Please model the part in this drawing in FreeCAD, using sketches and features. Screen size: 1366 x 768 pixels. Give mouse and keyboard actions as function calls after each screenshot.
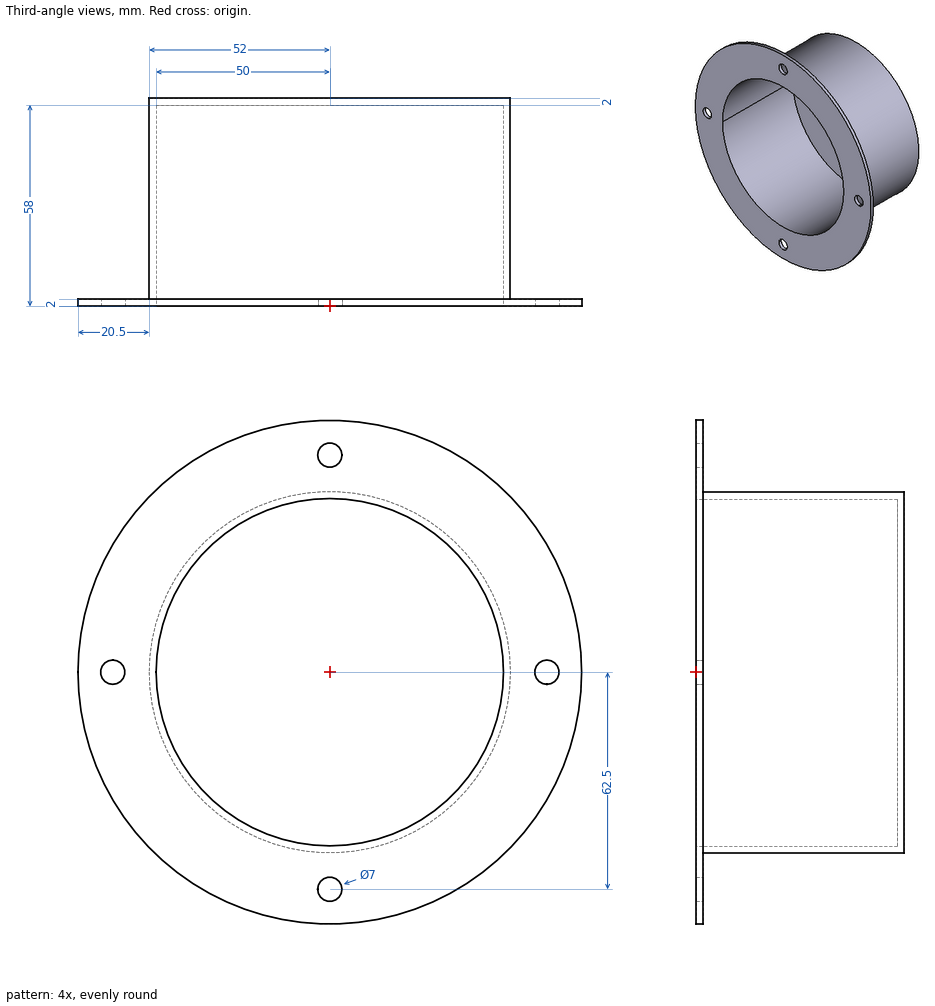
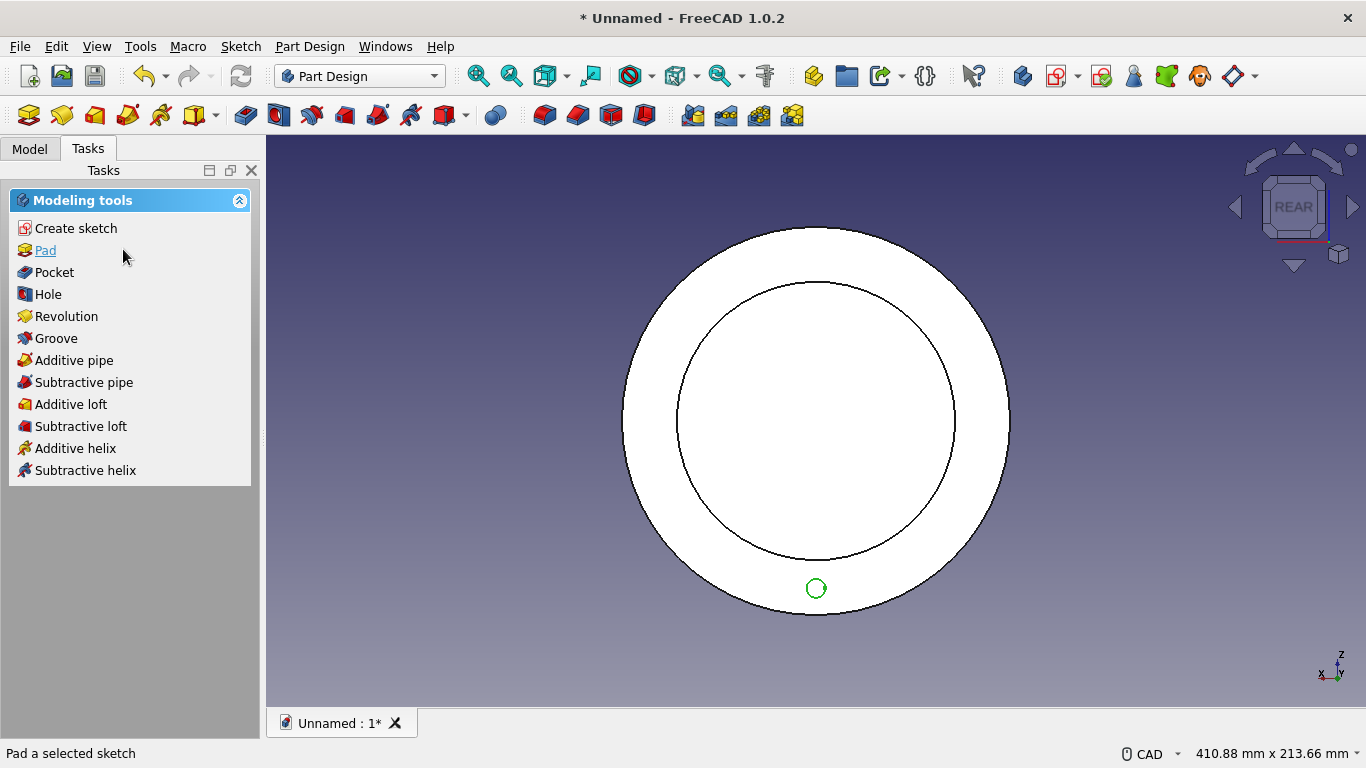
click(246, 116)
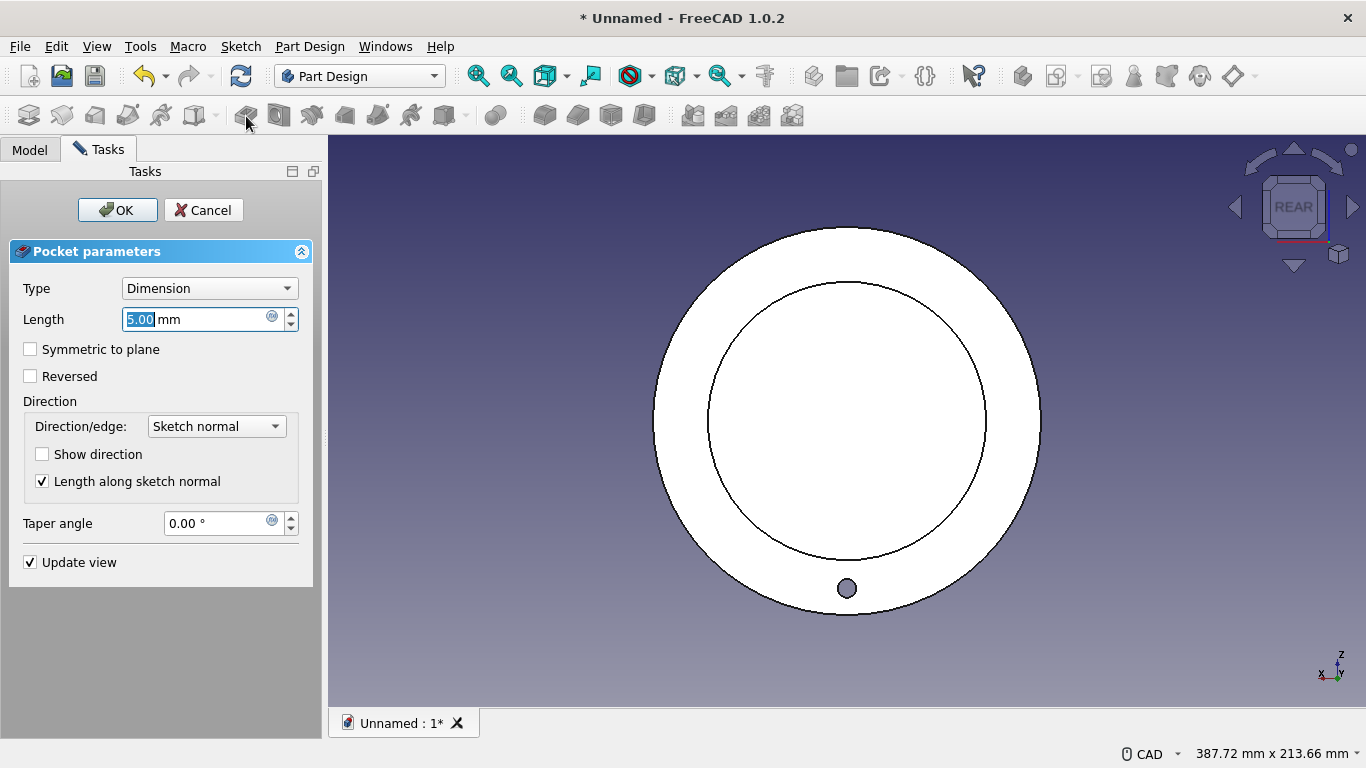
click(210, 288)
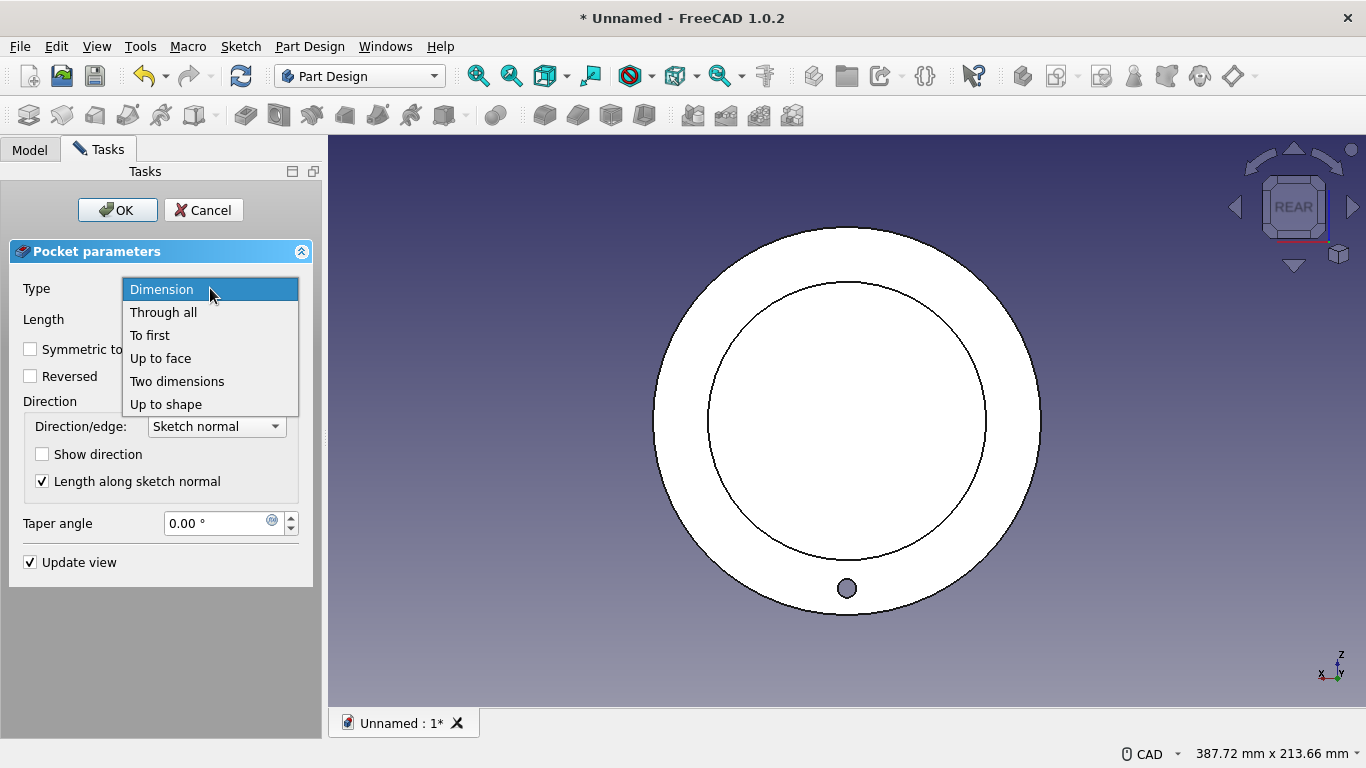
click(208, 312)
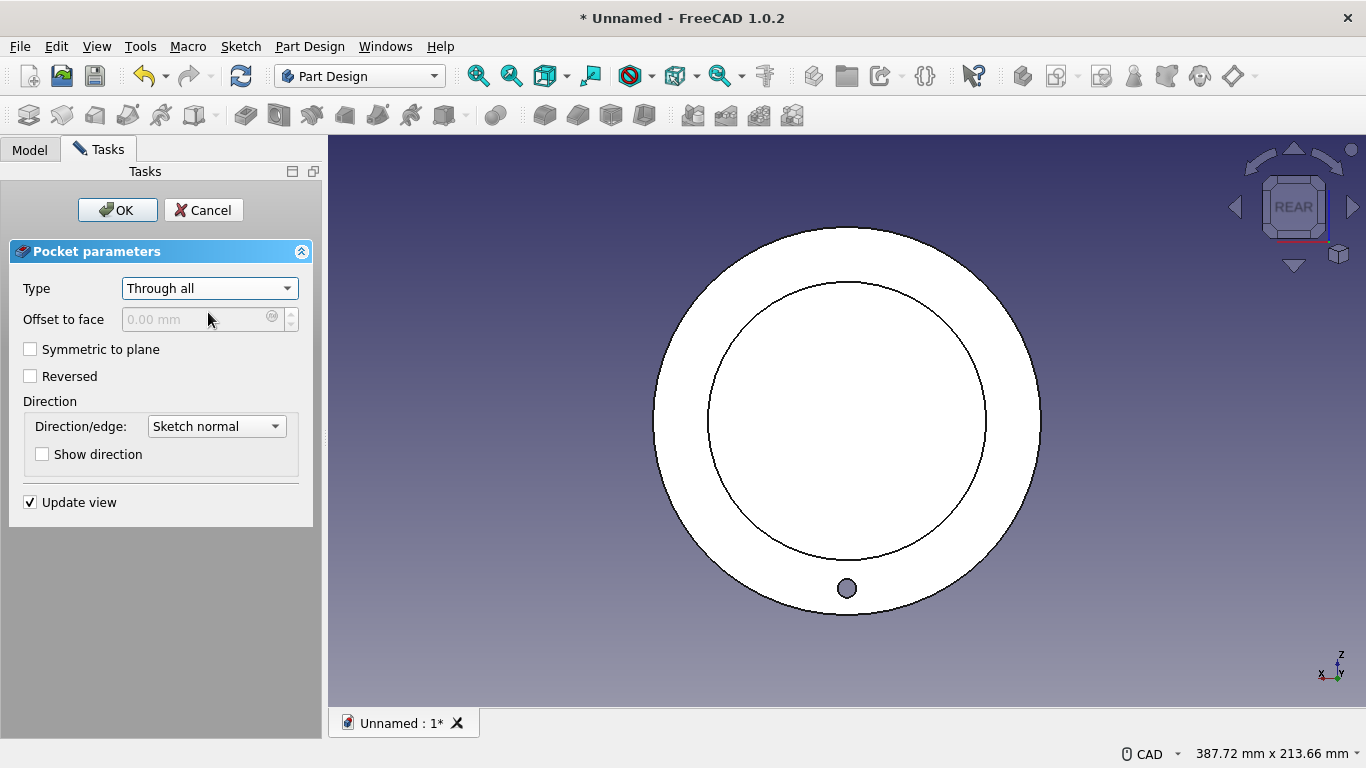
click(118, 210)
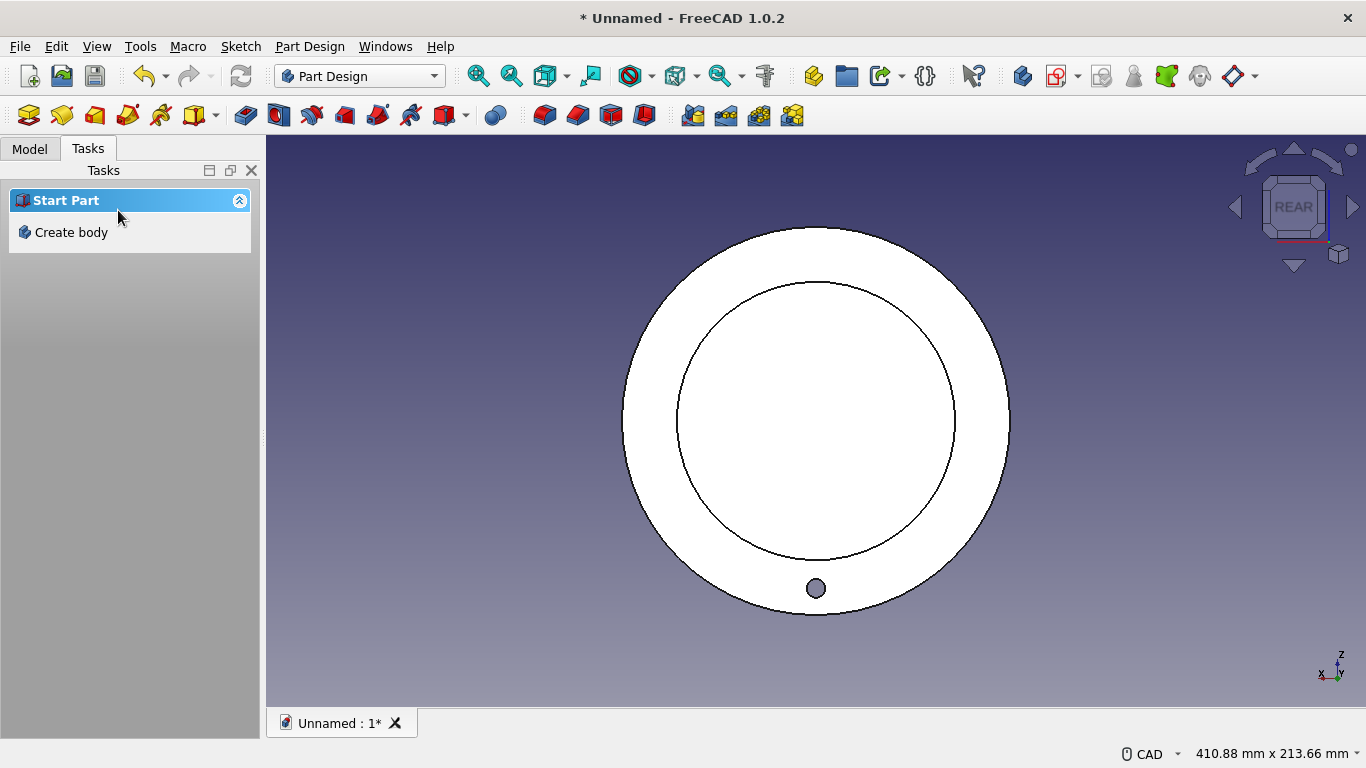
click(30, 148)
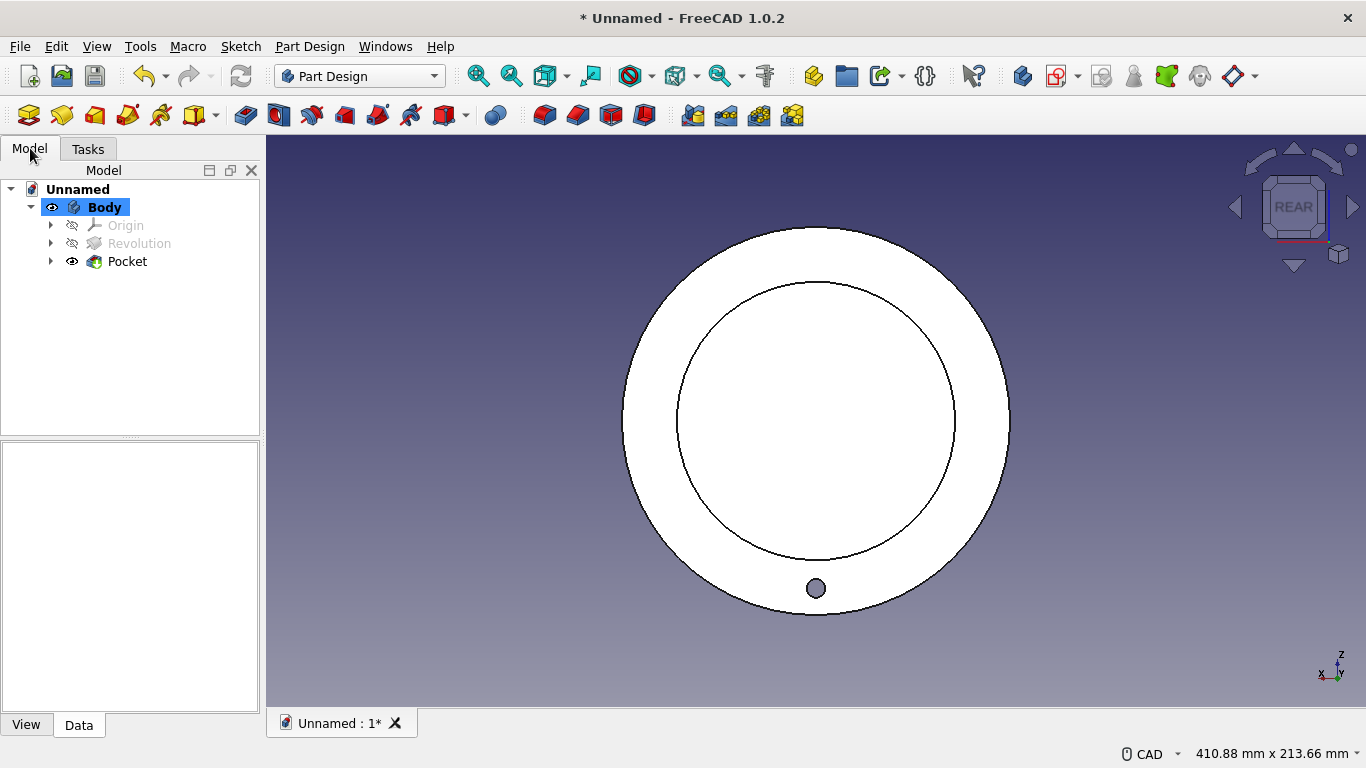
click(117, 261)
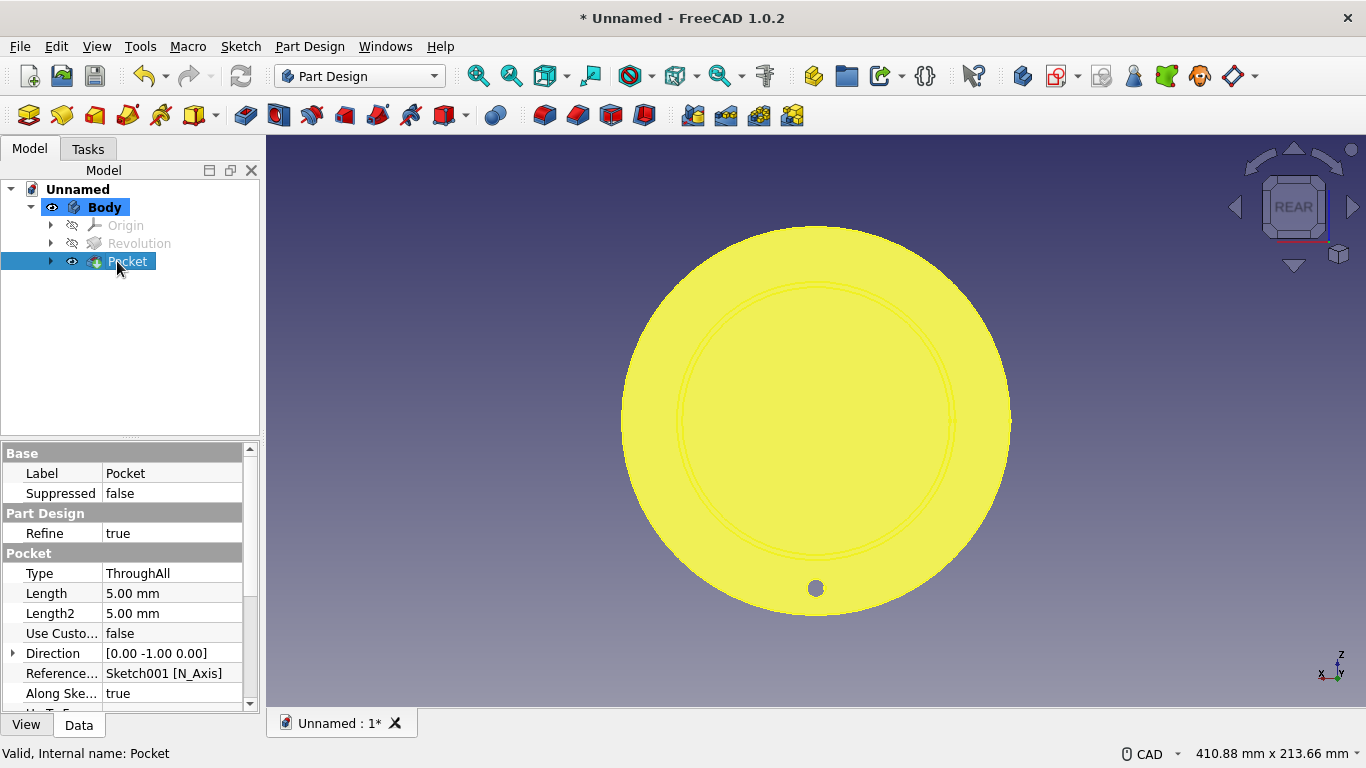
click(759, 116)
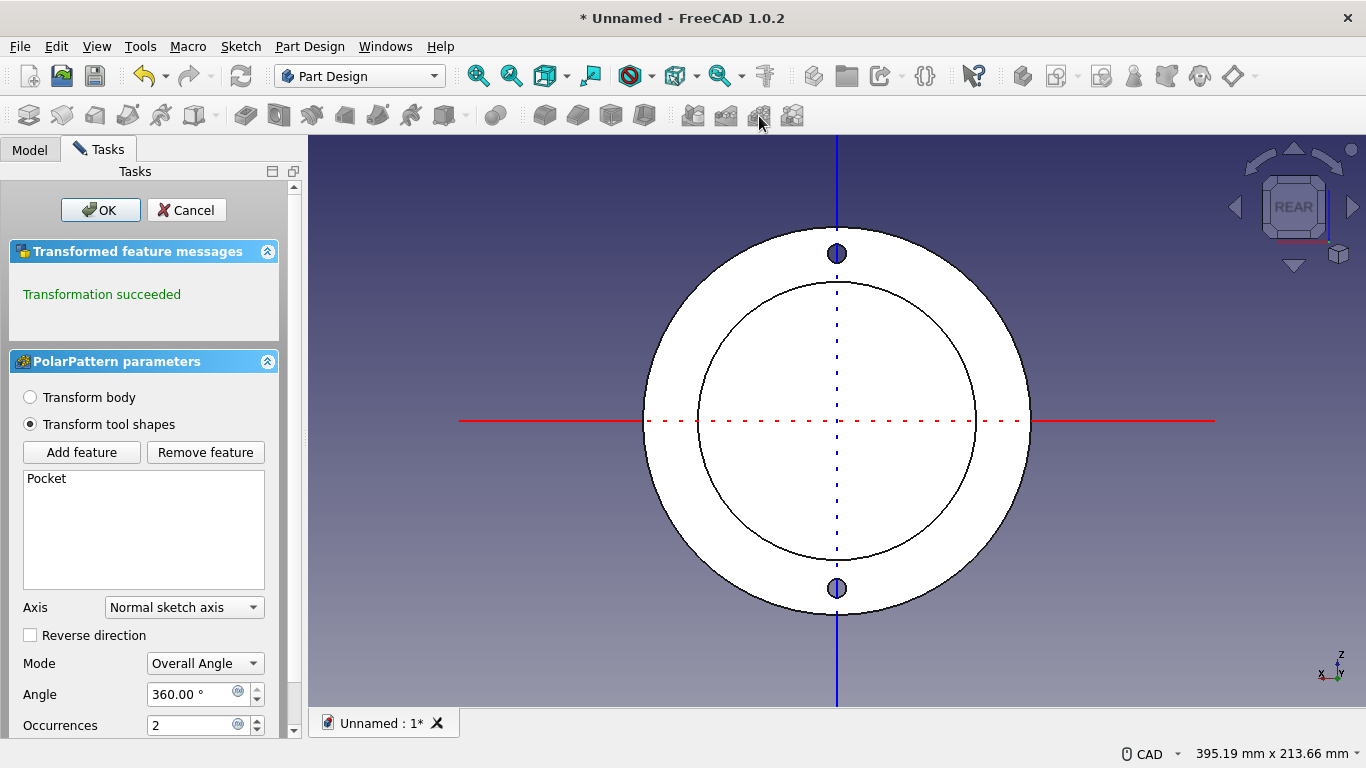
click(185, 608)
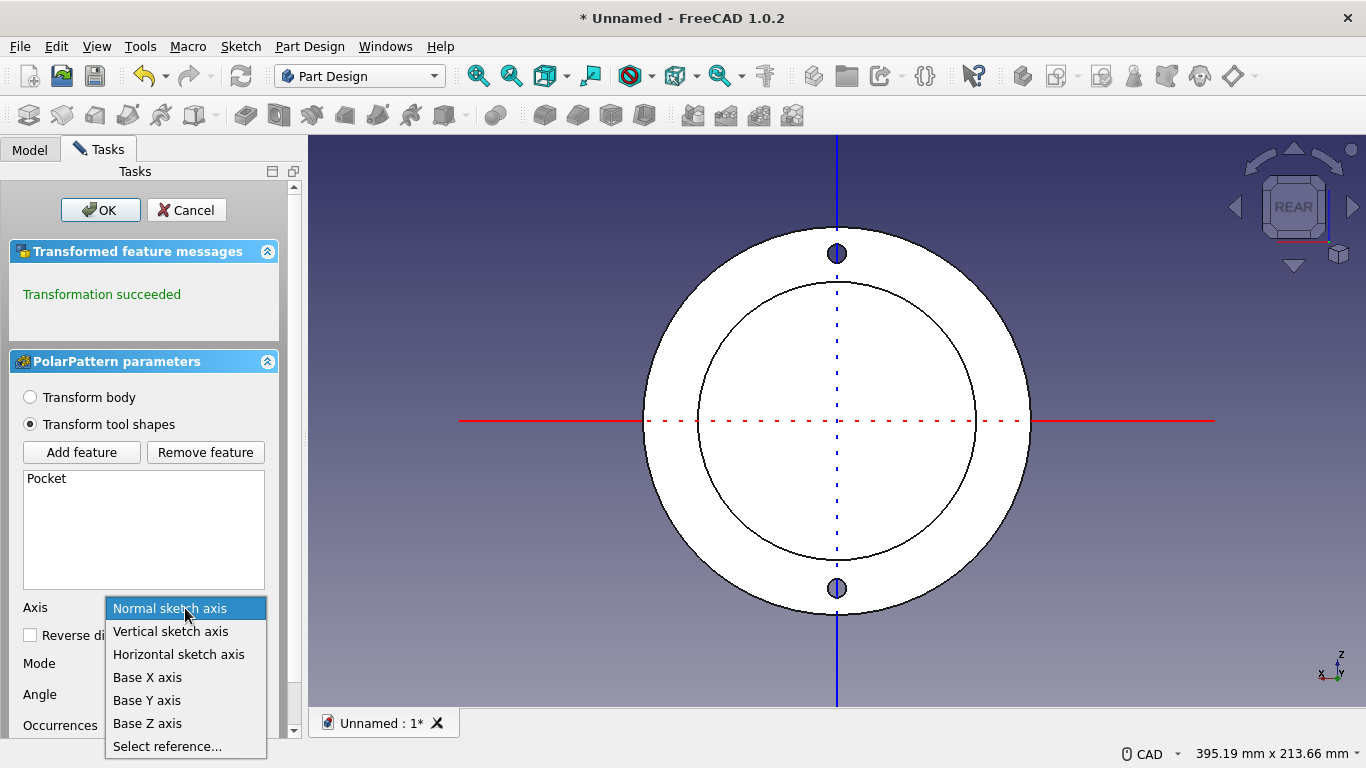
click(184, 700)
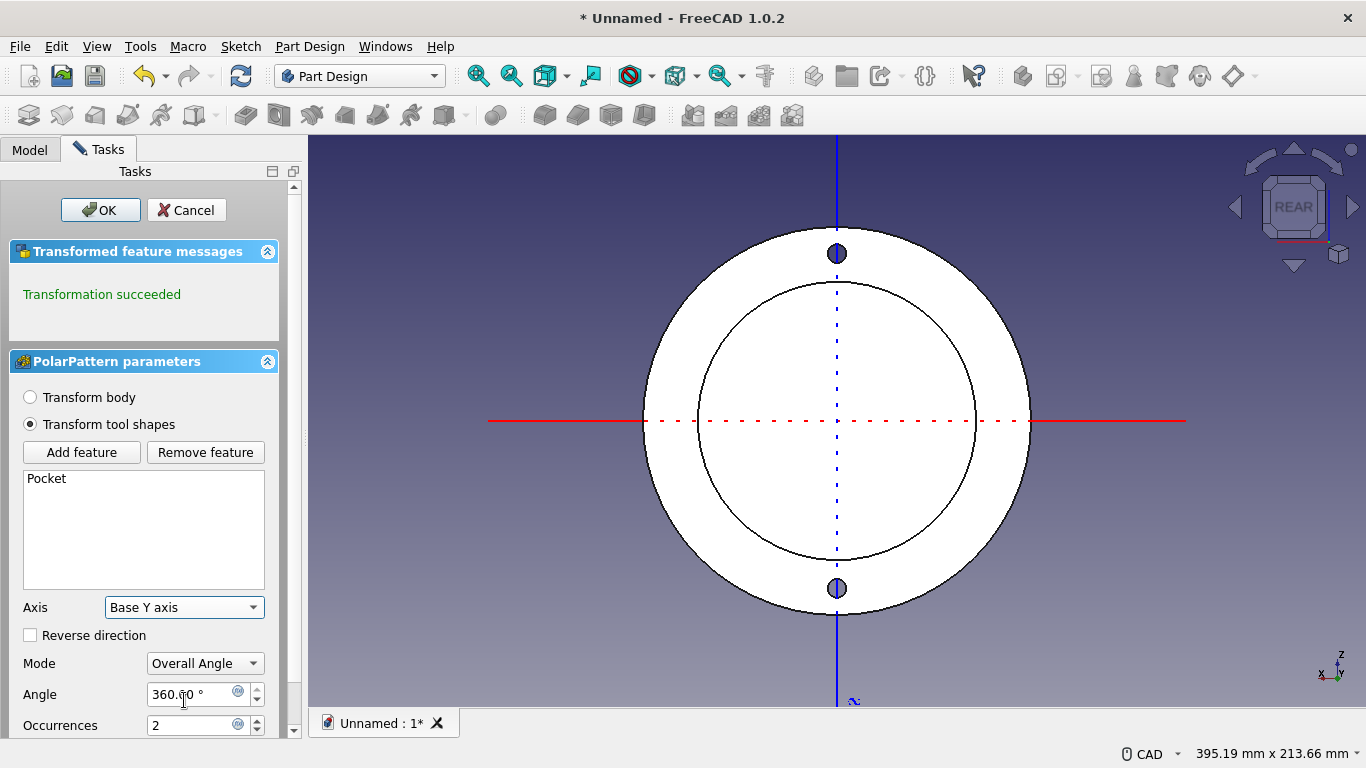
triple_click(199, 726)